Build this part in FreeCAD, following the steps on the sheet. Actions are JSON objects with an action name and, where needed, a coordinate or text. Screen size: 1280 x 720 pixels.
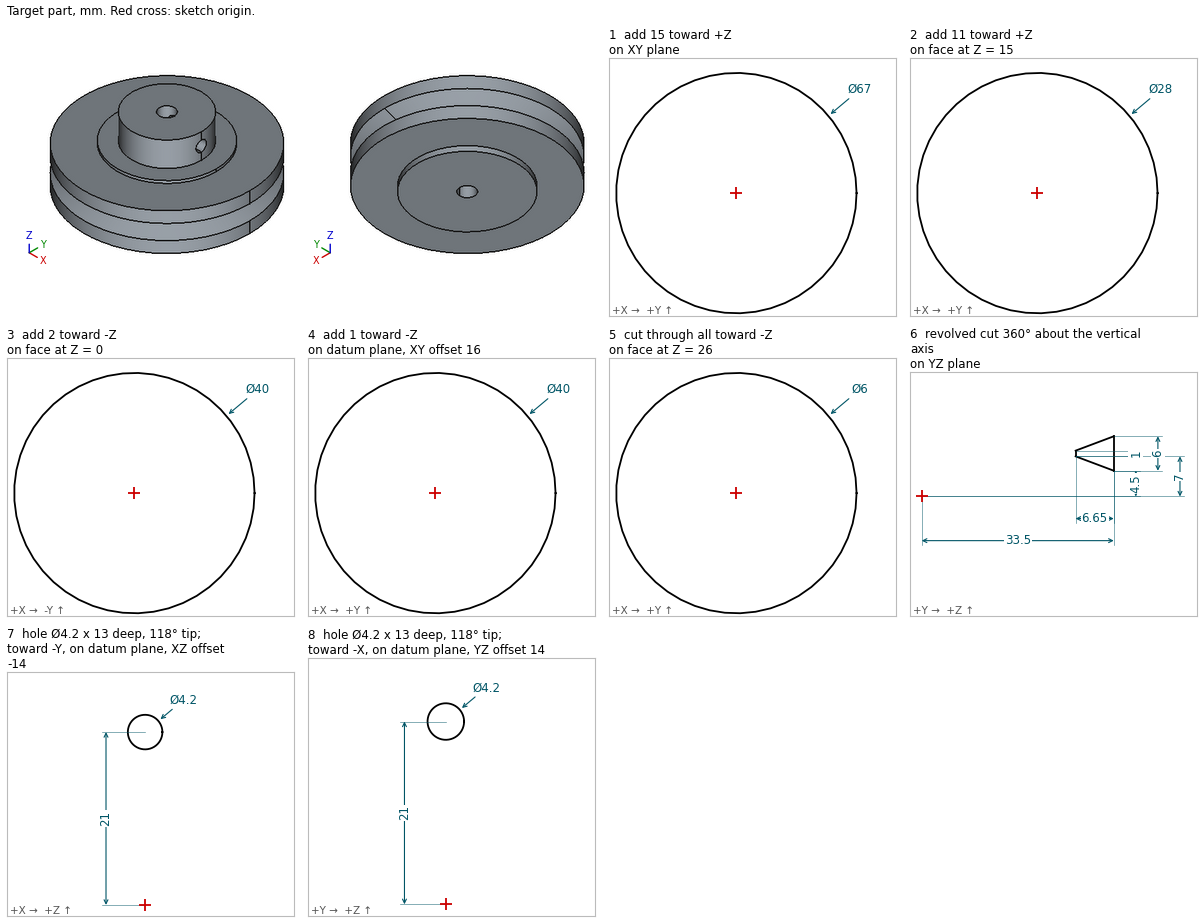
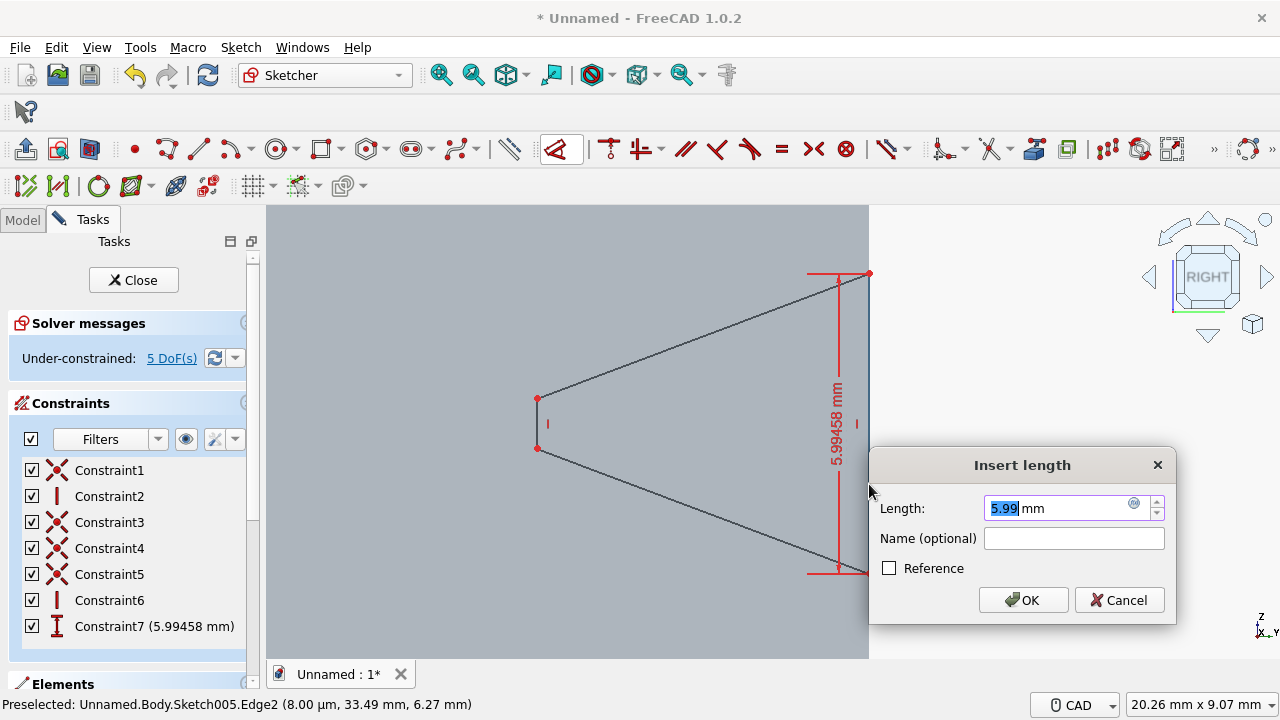
{"action": "type", "text": "6"}
{"action": "key", "text": "Return"}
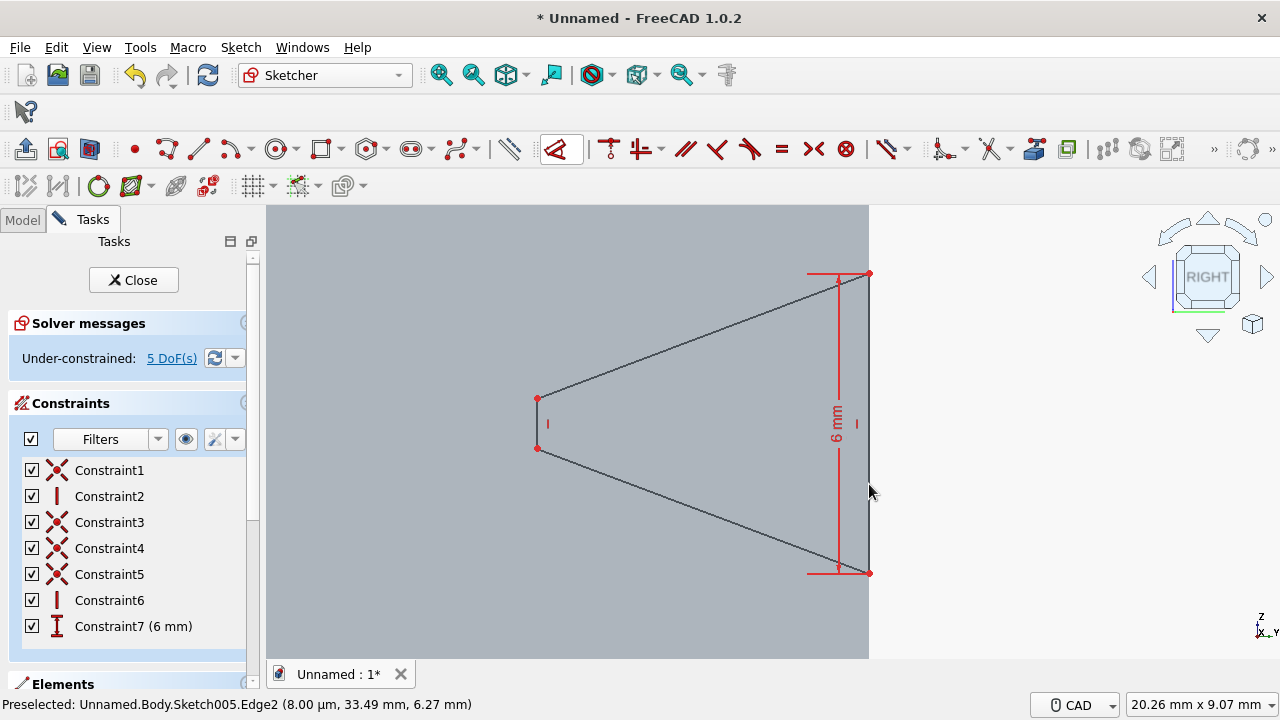
{"action": "left_click", "coordinate": [537, 414]}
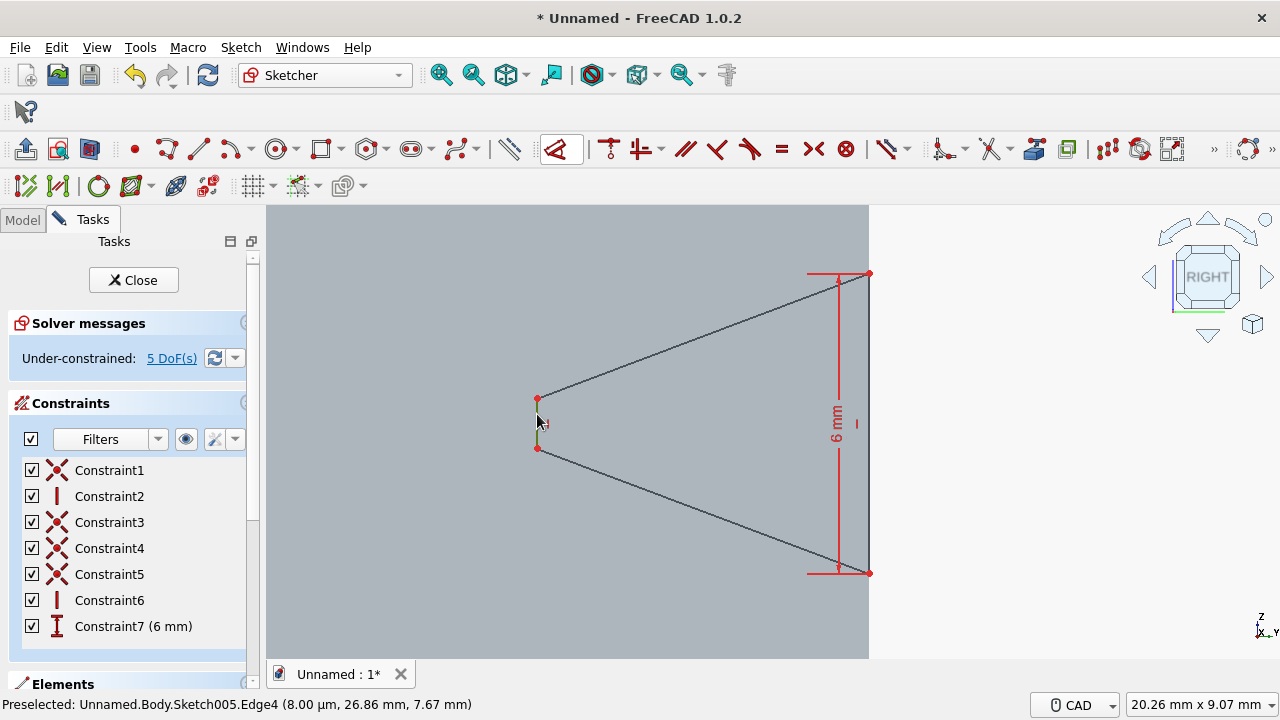
{"action": "key", "text": "i"}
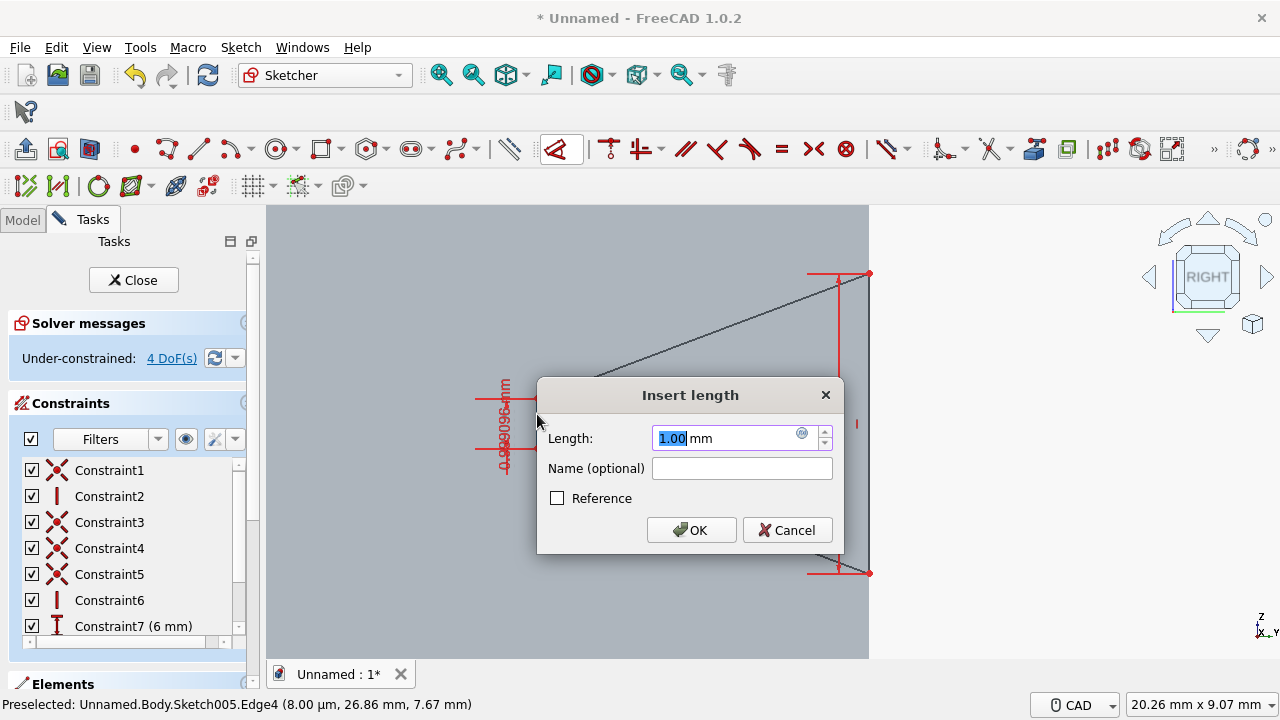
{"action": "type", "text": "1"}
{"action": "key", "text": "Return"}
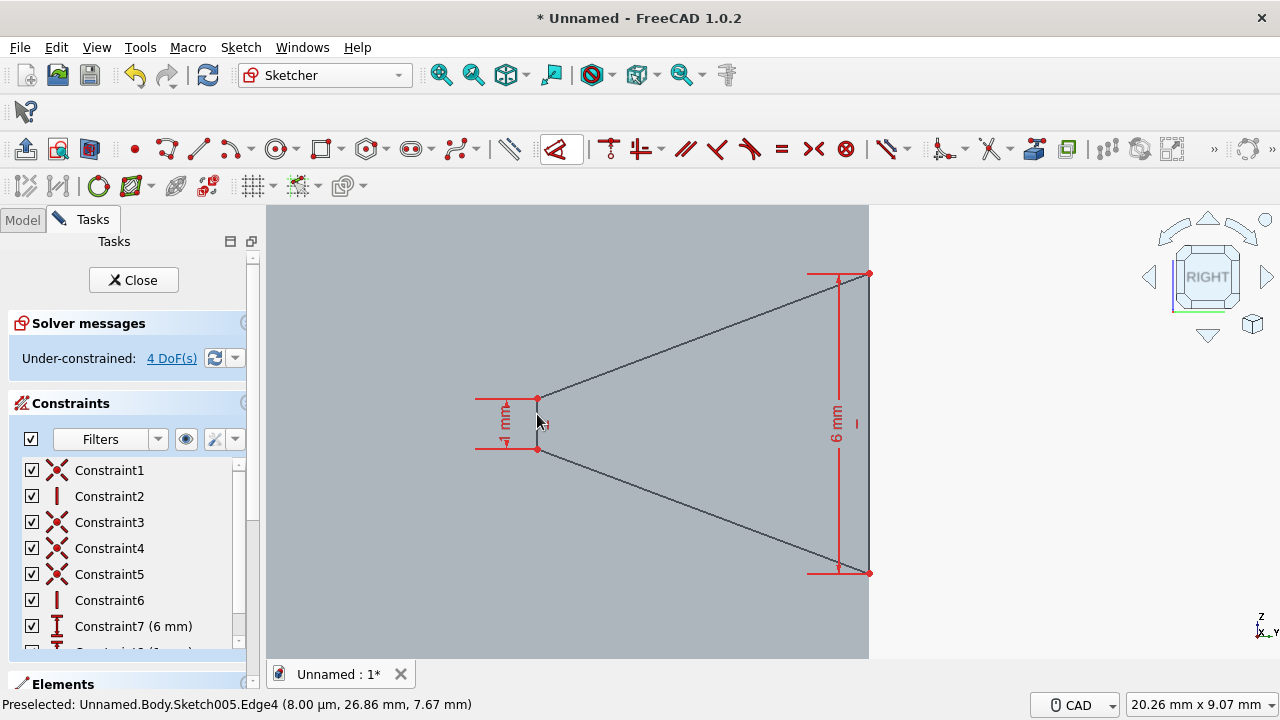
{"action": "left_click", "coordinate": [537, 449]}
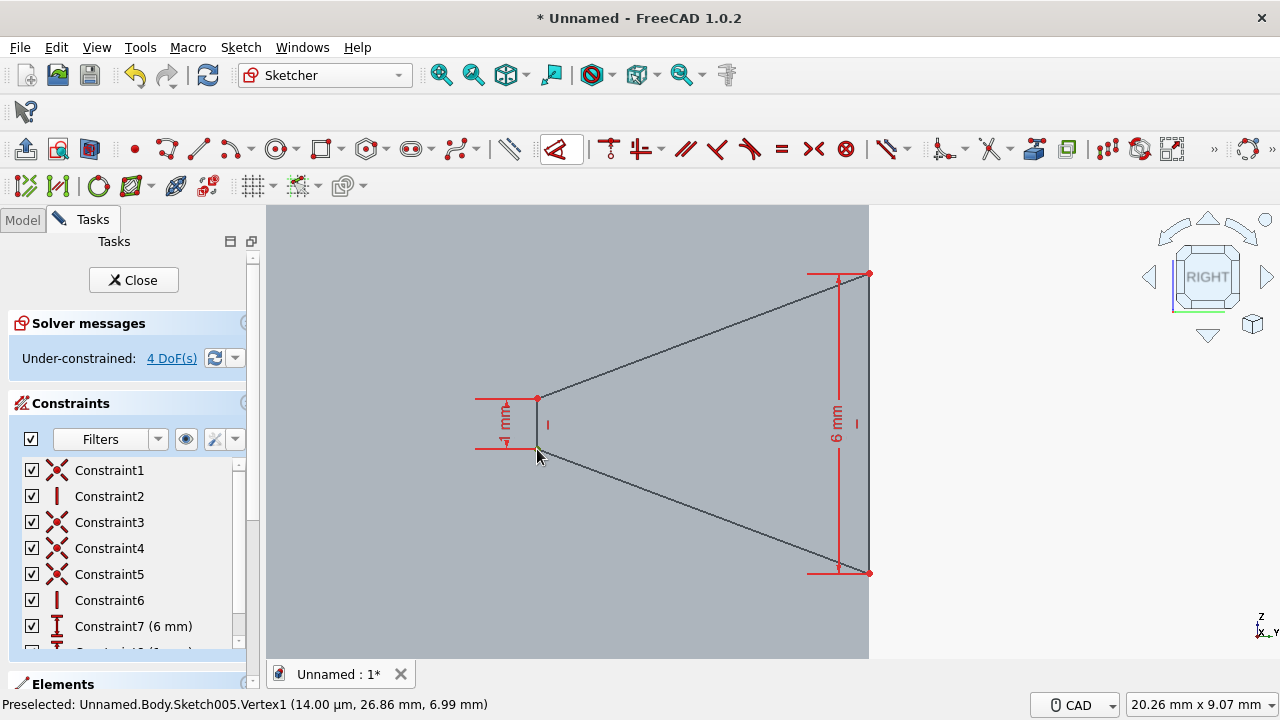
{"action": "key", "text": "i"}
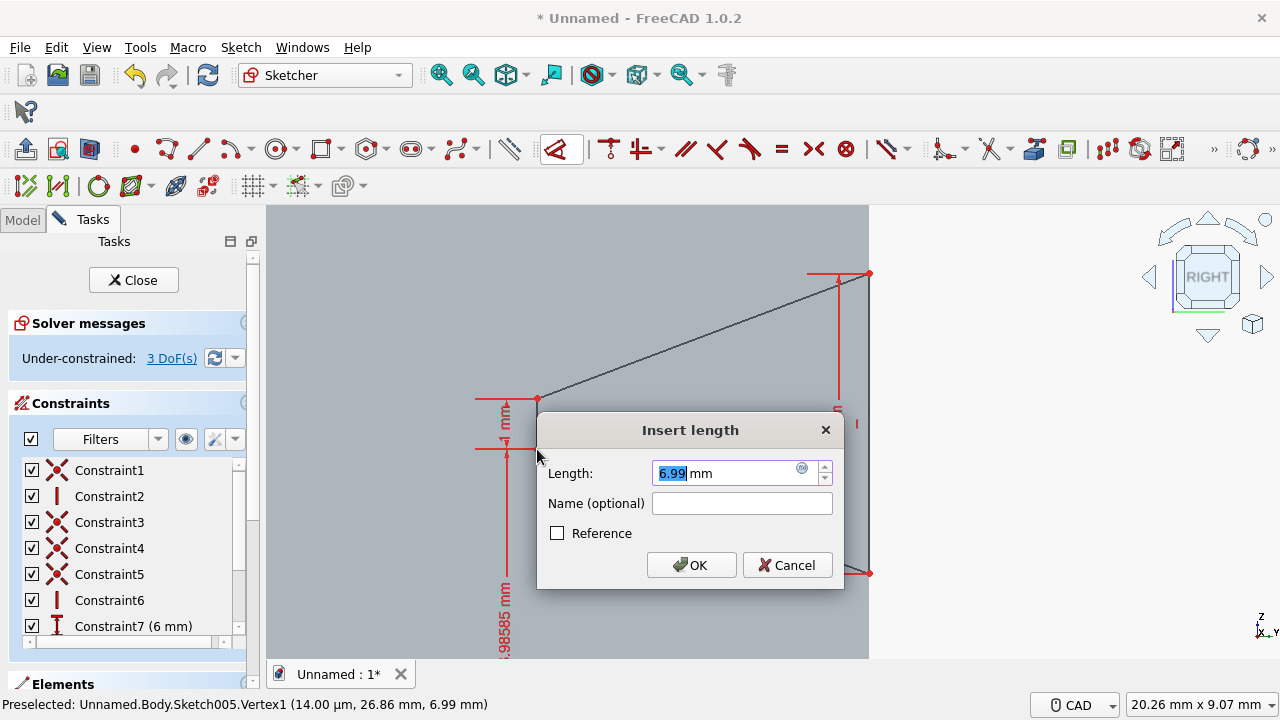
{"action": "type", "text": "7"}
{"action": "key", "text": "Return"}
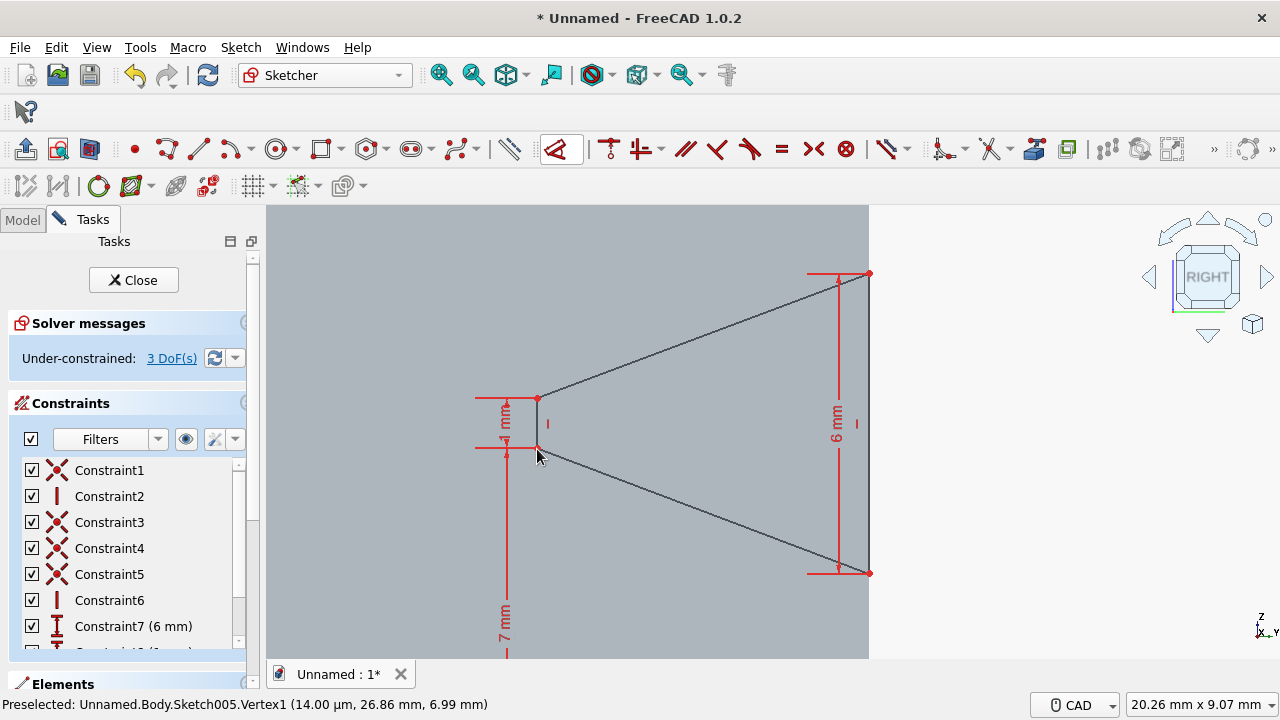
{"action": "left_click", "coordinate": [869, 574]}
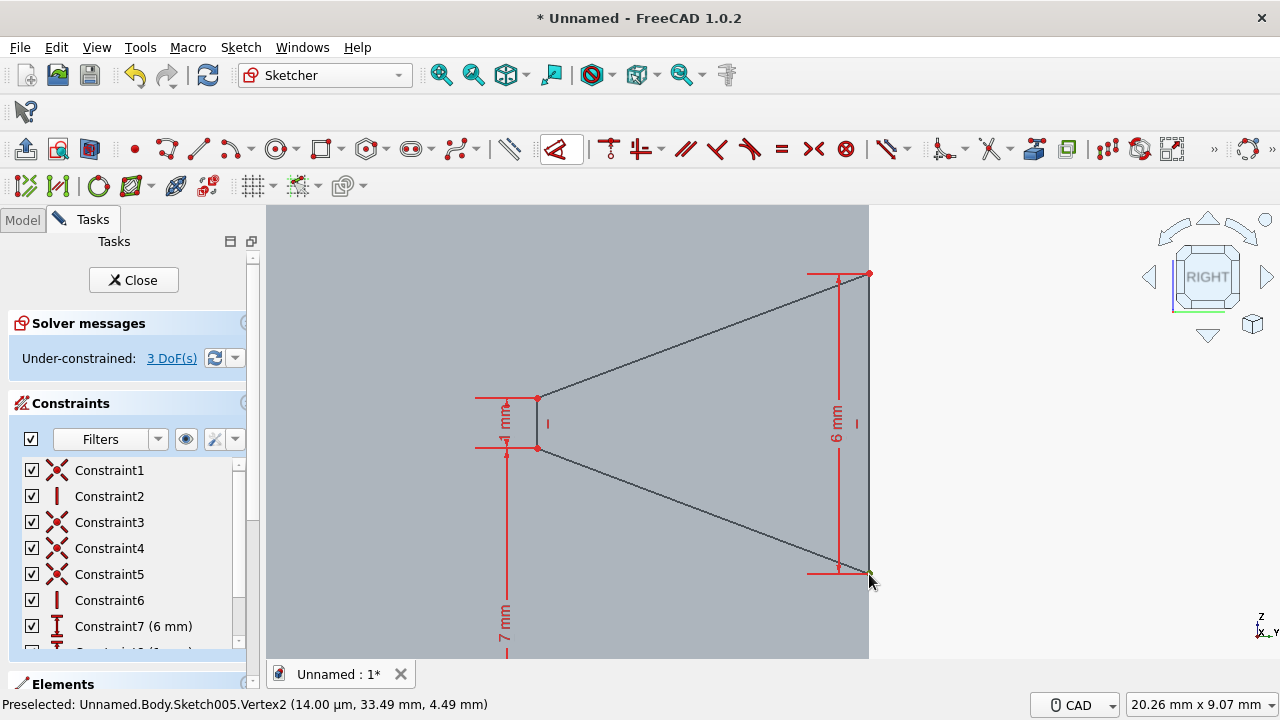
{"action": "key", "text": "i"}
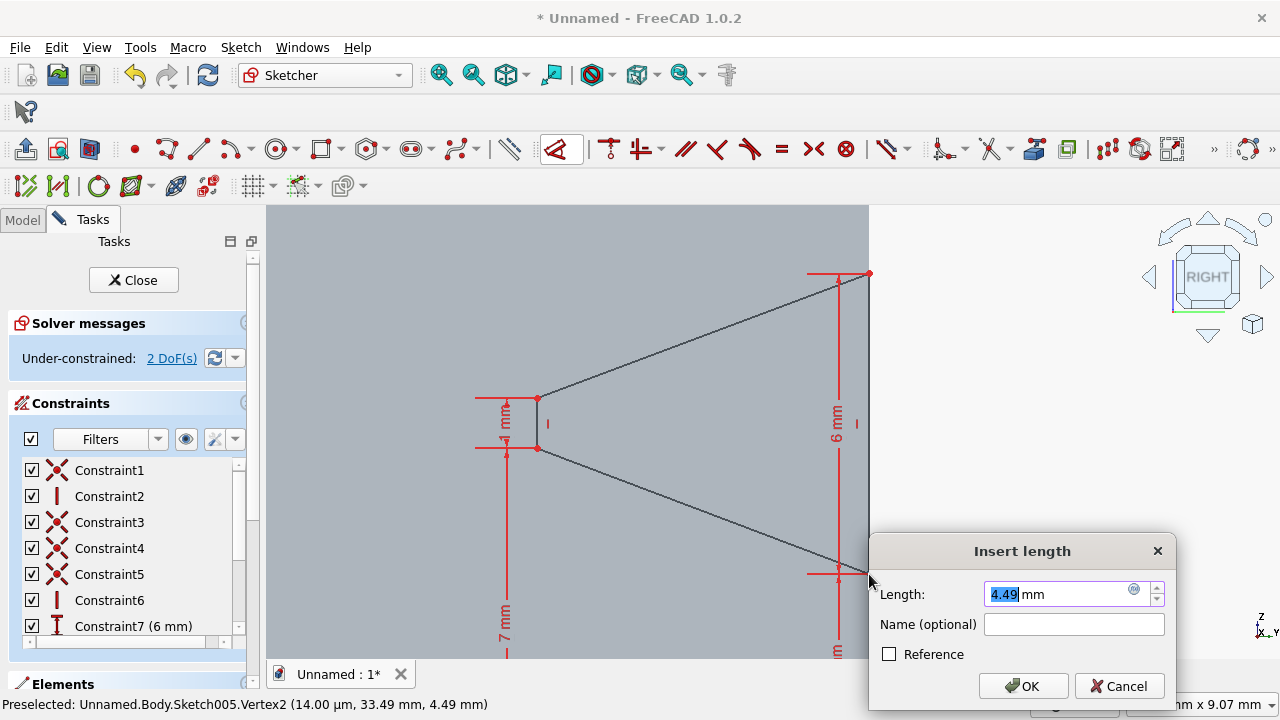
{"action": "type", "text": "4.5"}
{"action": "key", "text": "Return"}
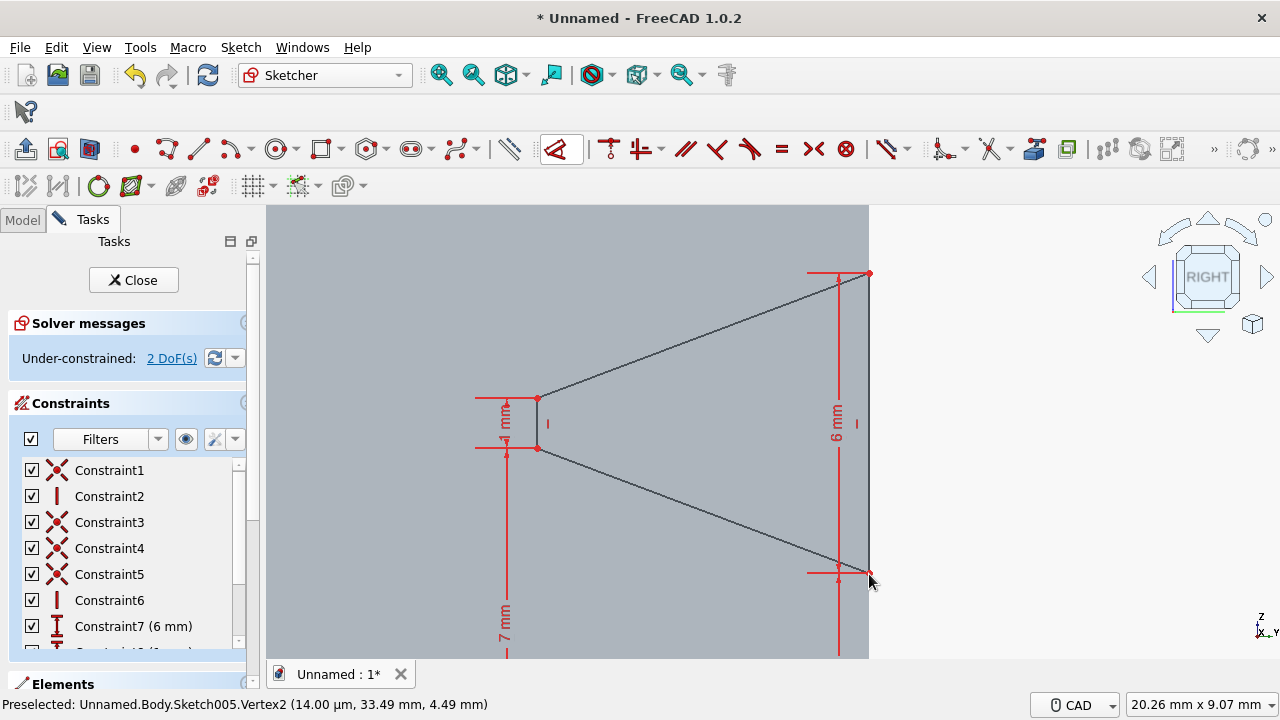
{"action": "left_click", "coordinate": [869, 573]}